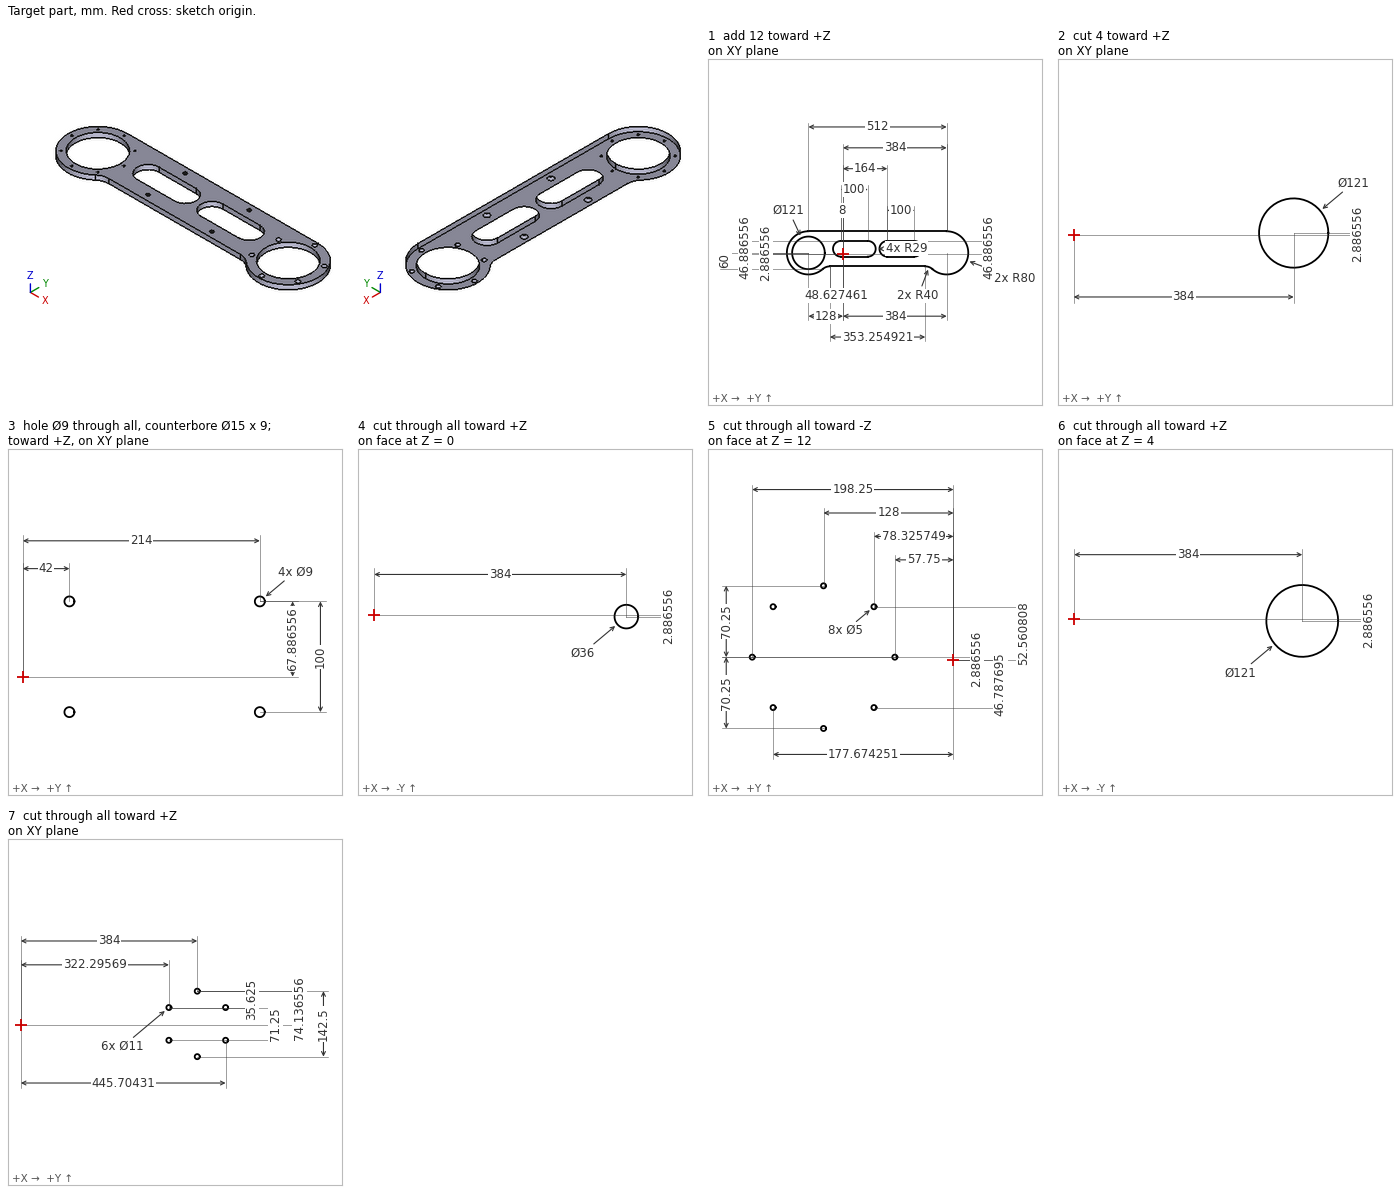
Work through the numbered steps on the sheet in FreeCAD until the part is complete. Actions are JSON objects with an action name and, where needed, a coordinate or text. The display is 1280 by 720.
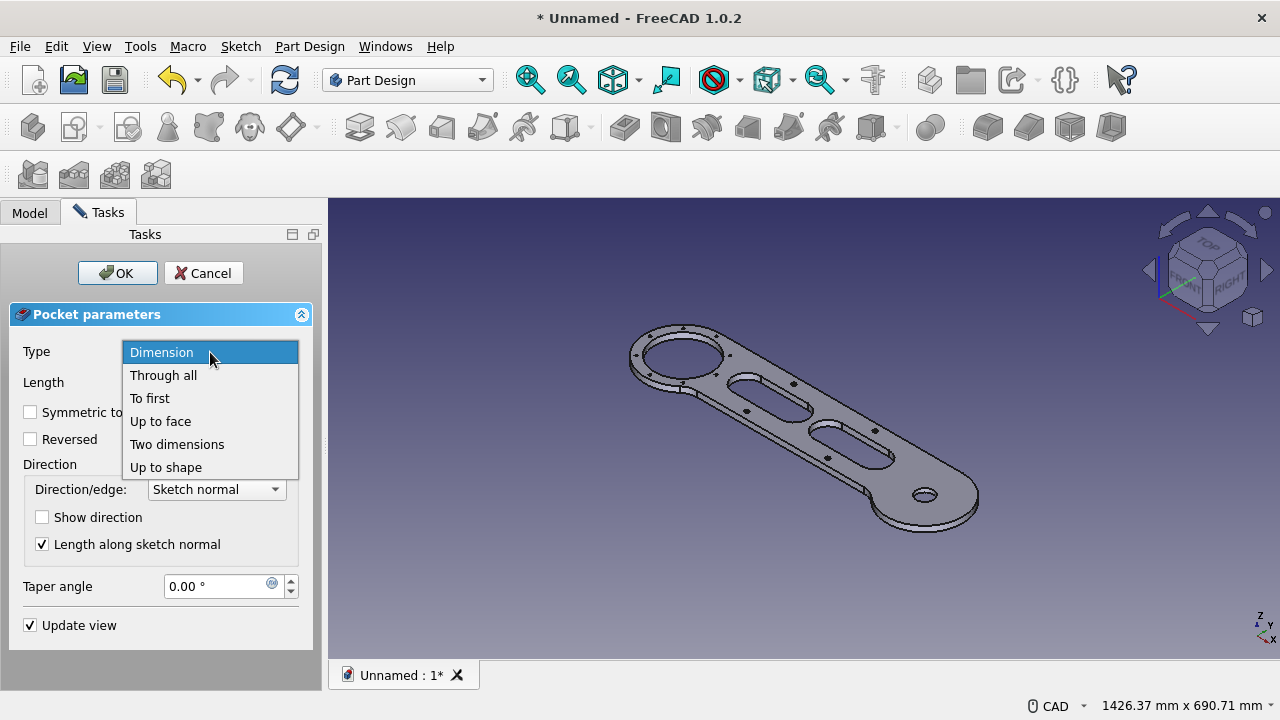
{"action": "left_click", "coordinate": [208, 376]}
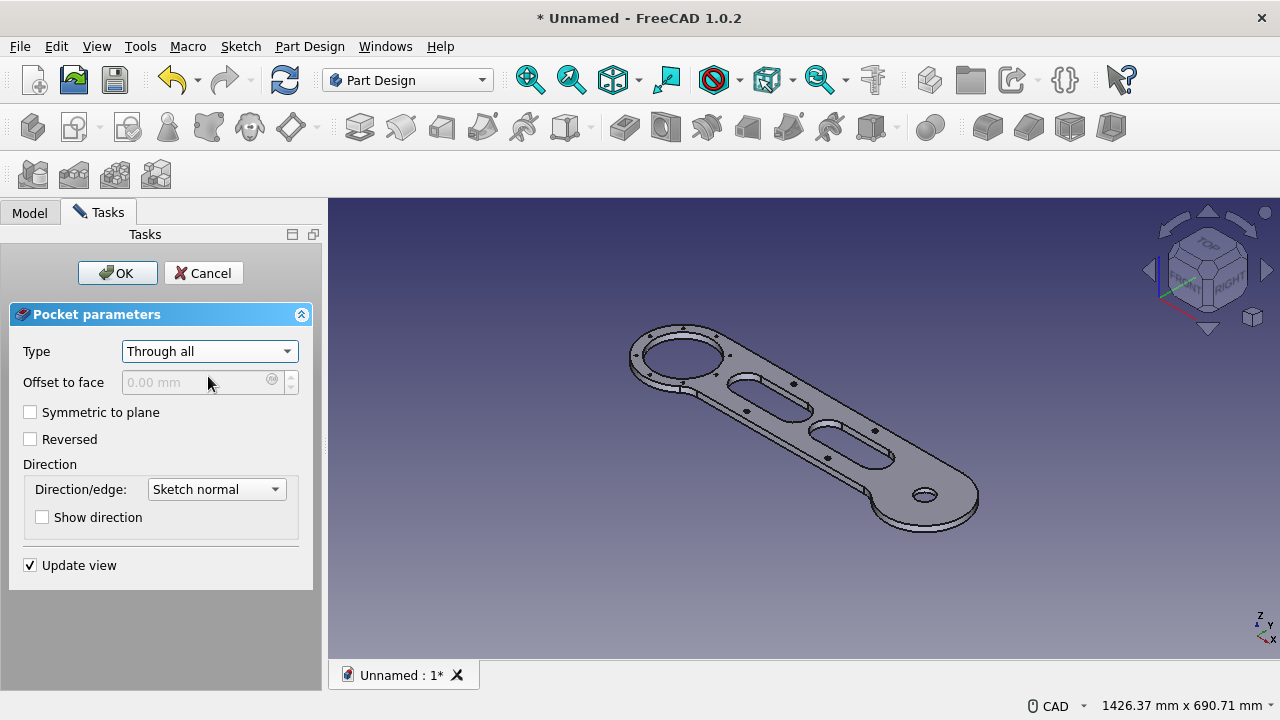
{"action": "left_click", "coordinate": [118, 273]}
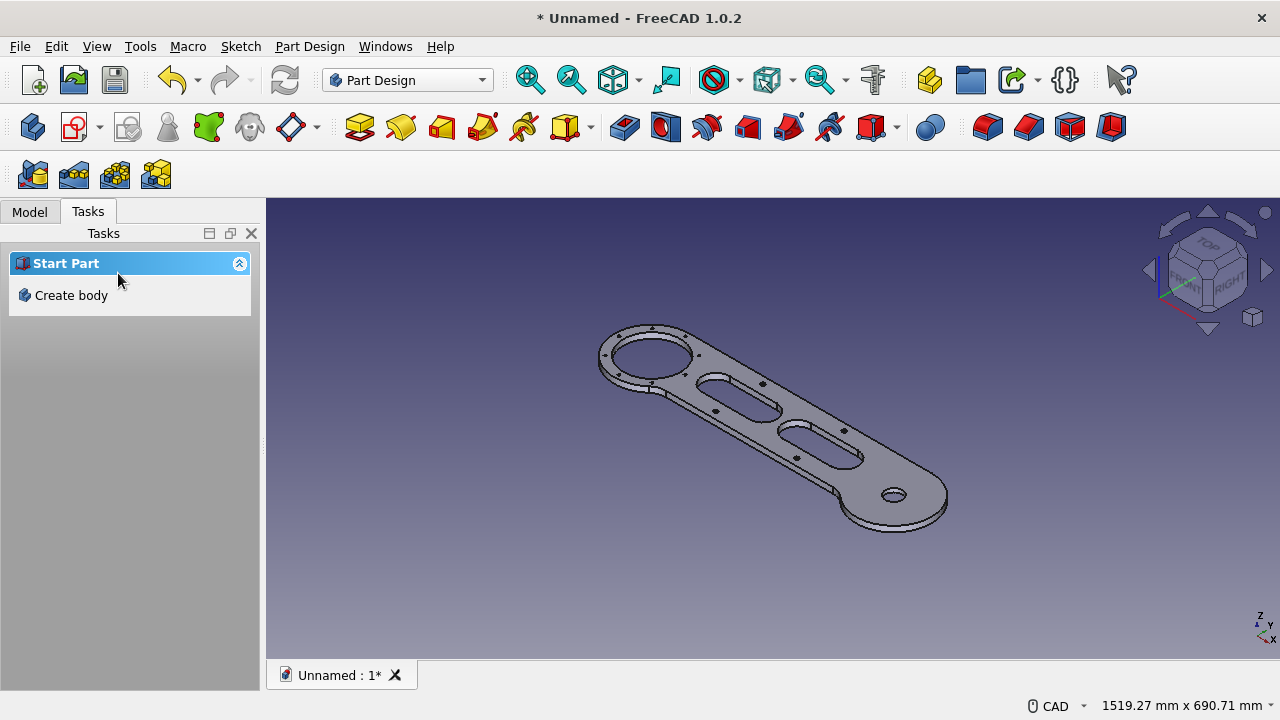
{"action": "key", "text": "5"}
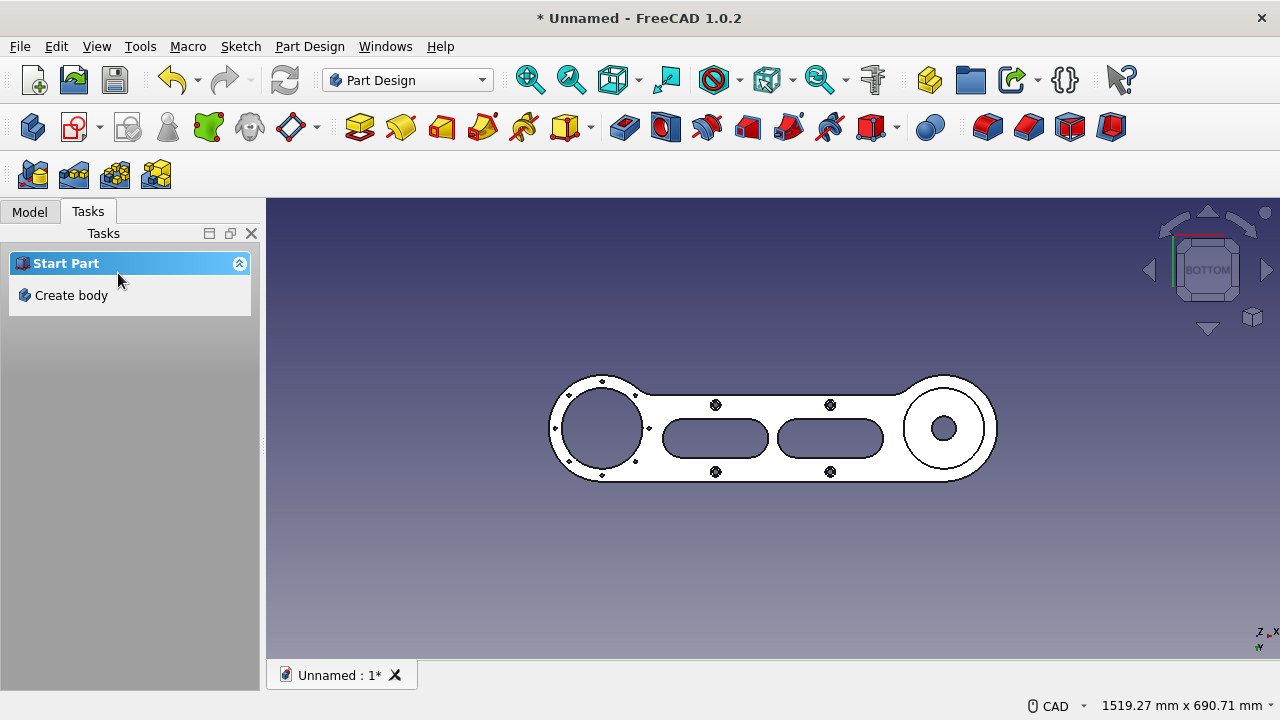
{"action": "left_click", "coordinate": [531, 80]}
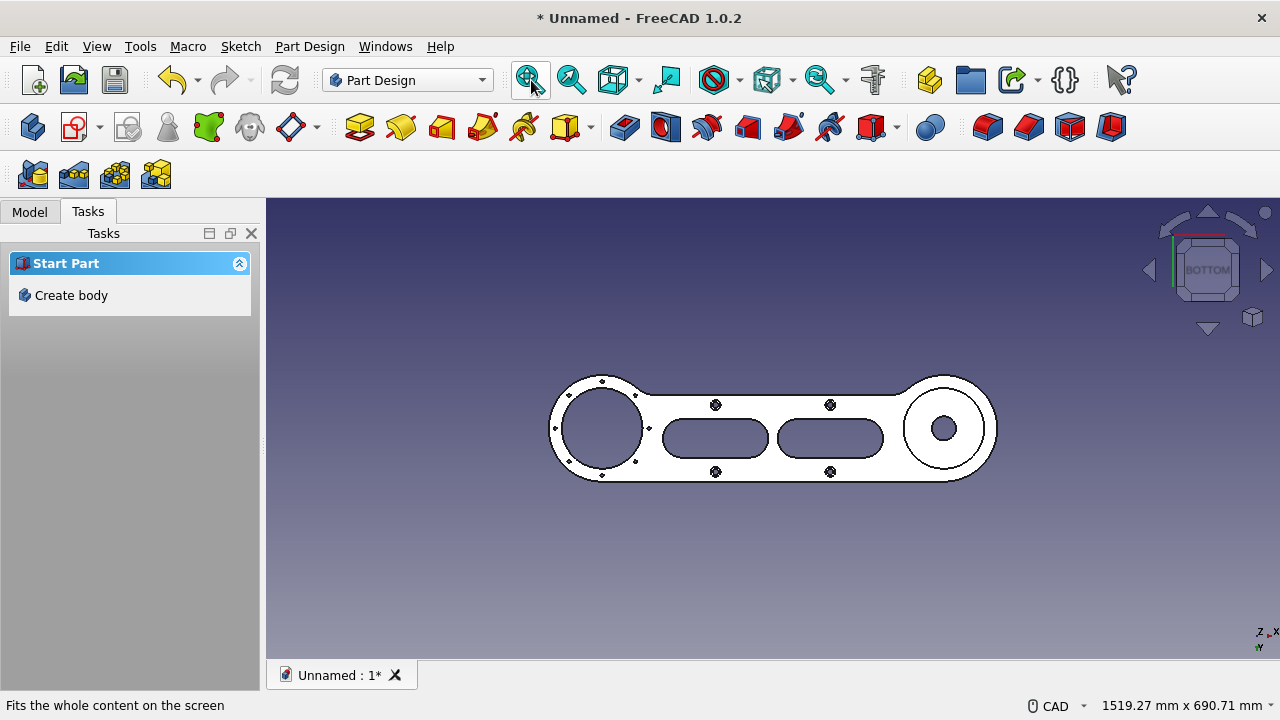
{"action": "left_click", "coordinate": [955, 450]}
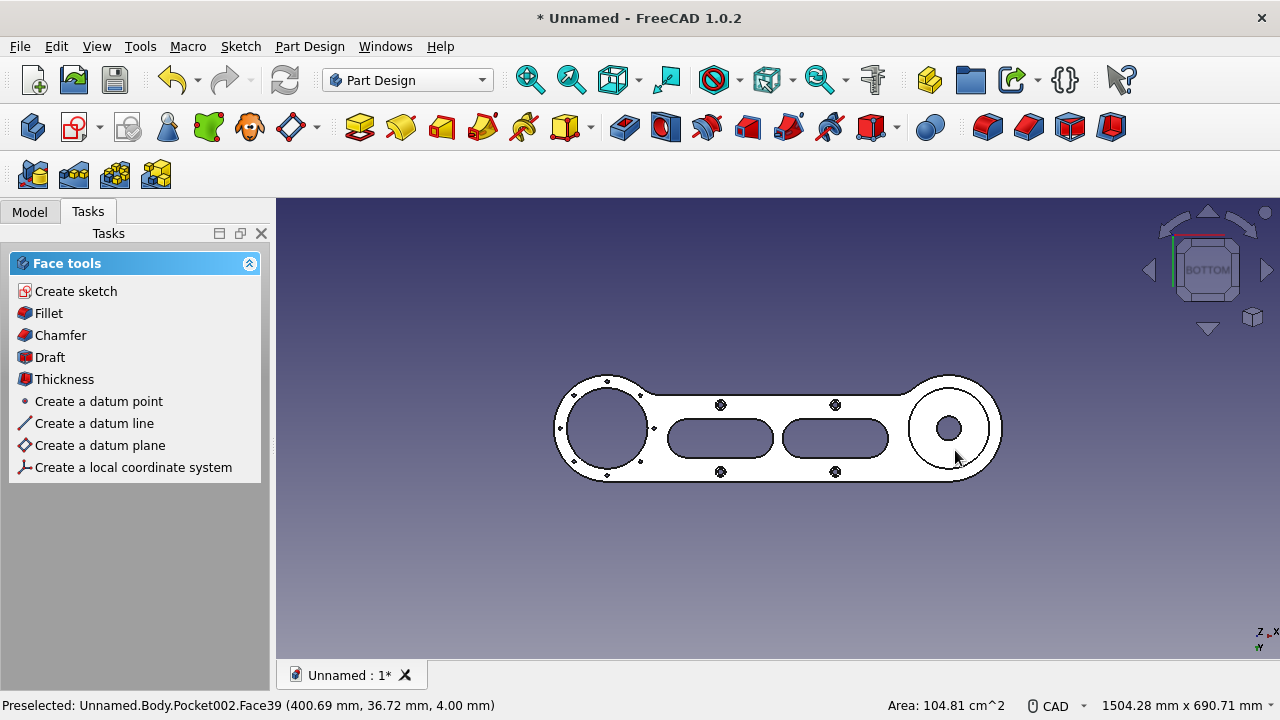
{"action": "left_click", "coordinate": [74, 128]}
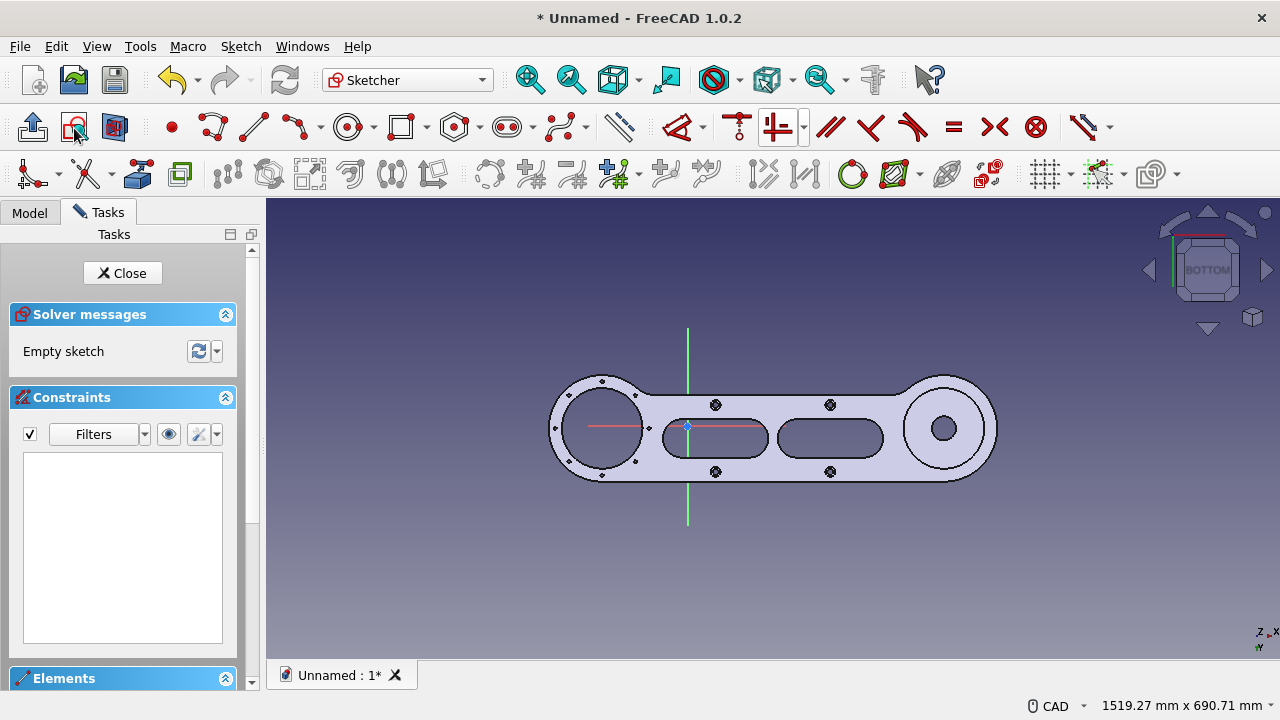
{"action": "scroll", "coordinate": [1047, 428], "scroll_direction": "up", "scroll_amount": 6}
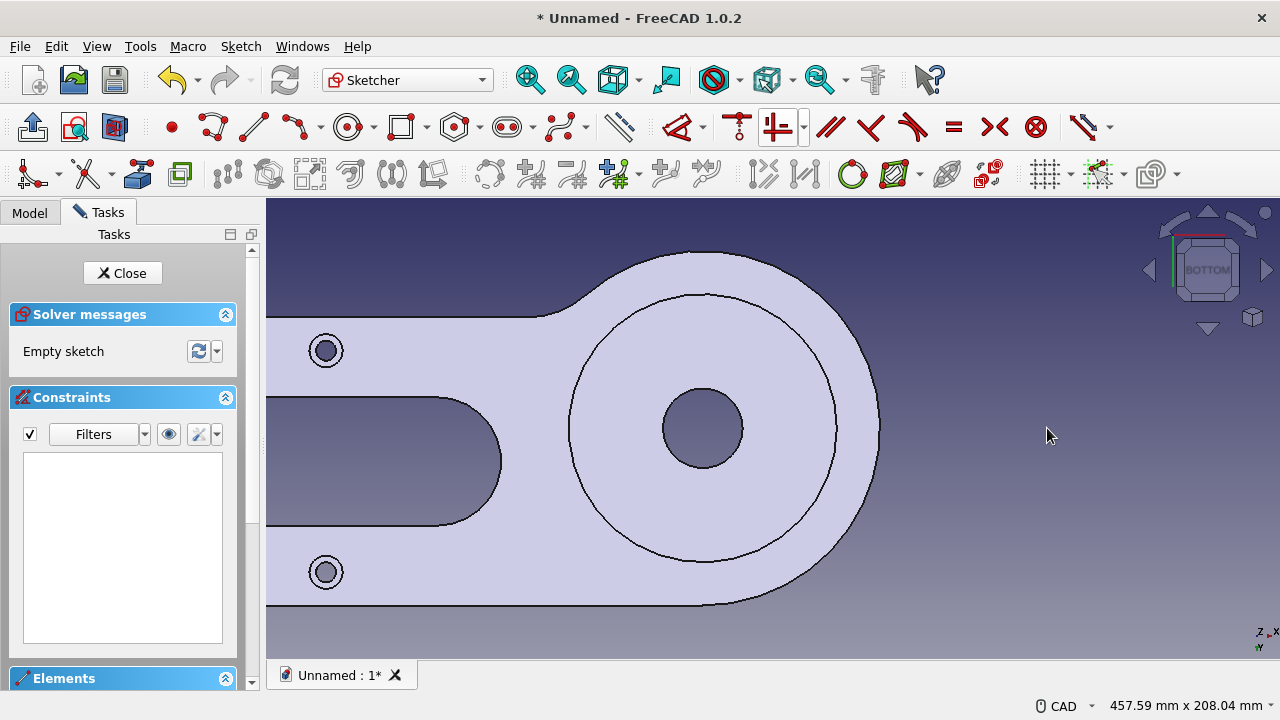
{"action": "left_click", "coordinate": [348, 128]}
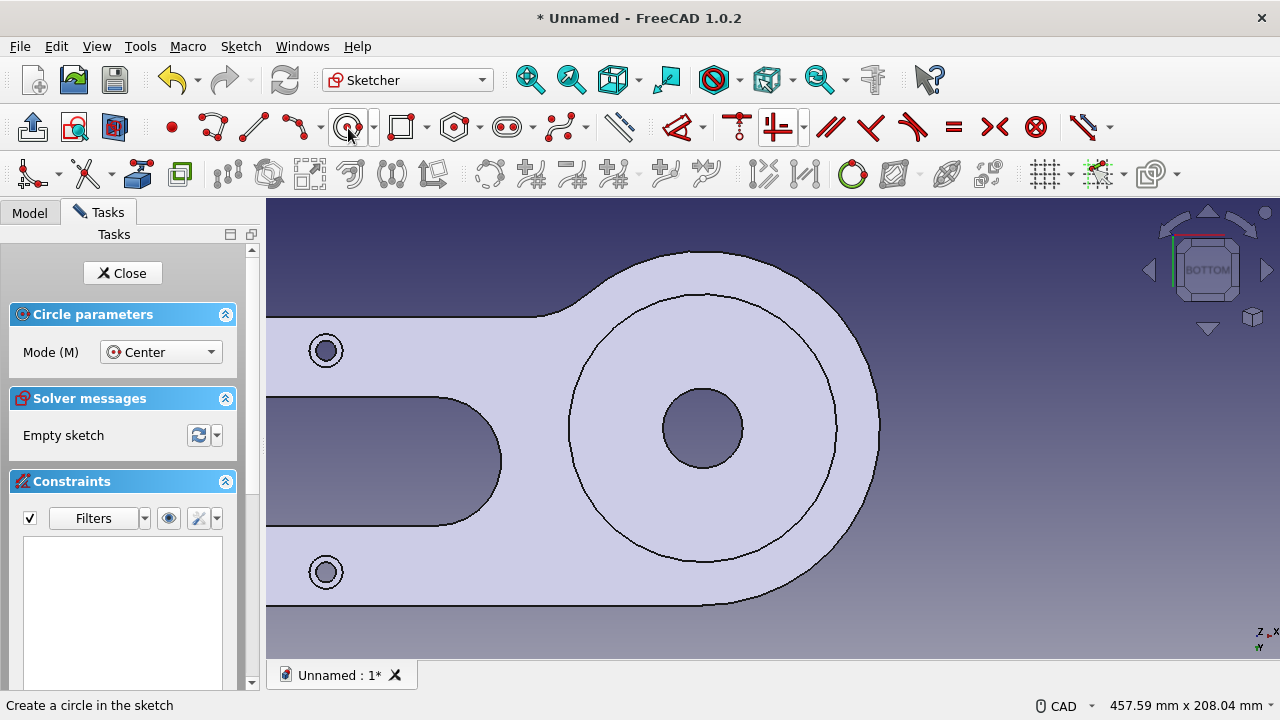
{"action": "scroll", "coordinate": [703, 428], "scroll_direction": "up", "scroll_amount": 5}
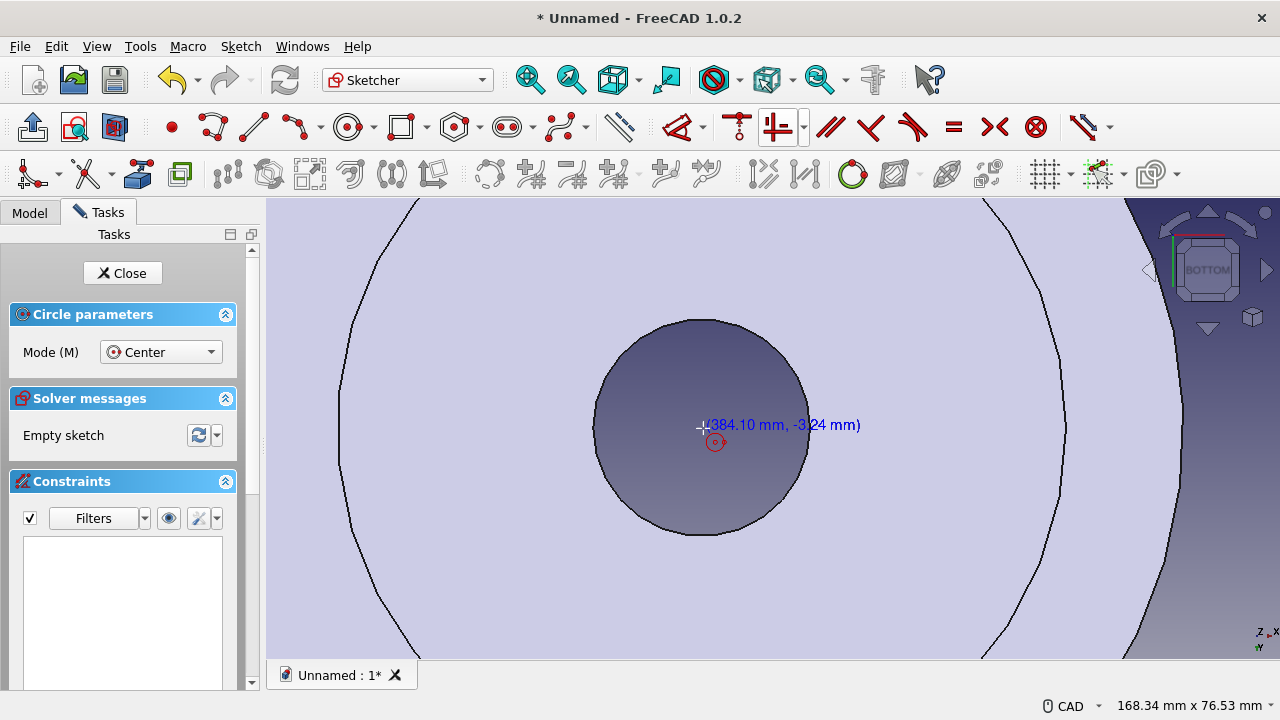
{"action": "left_click", "coordinate": [702, 428]}